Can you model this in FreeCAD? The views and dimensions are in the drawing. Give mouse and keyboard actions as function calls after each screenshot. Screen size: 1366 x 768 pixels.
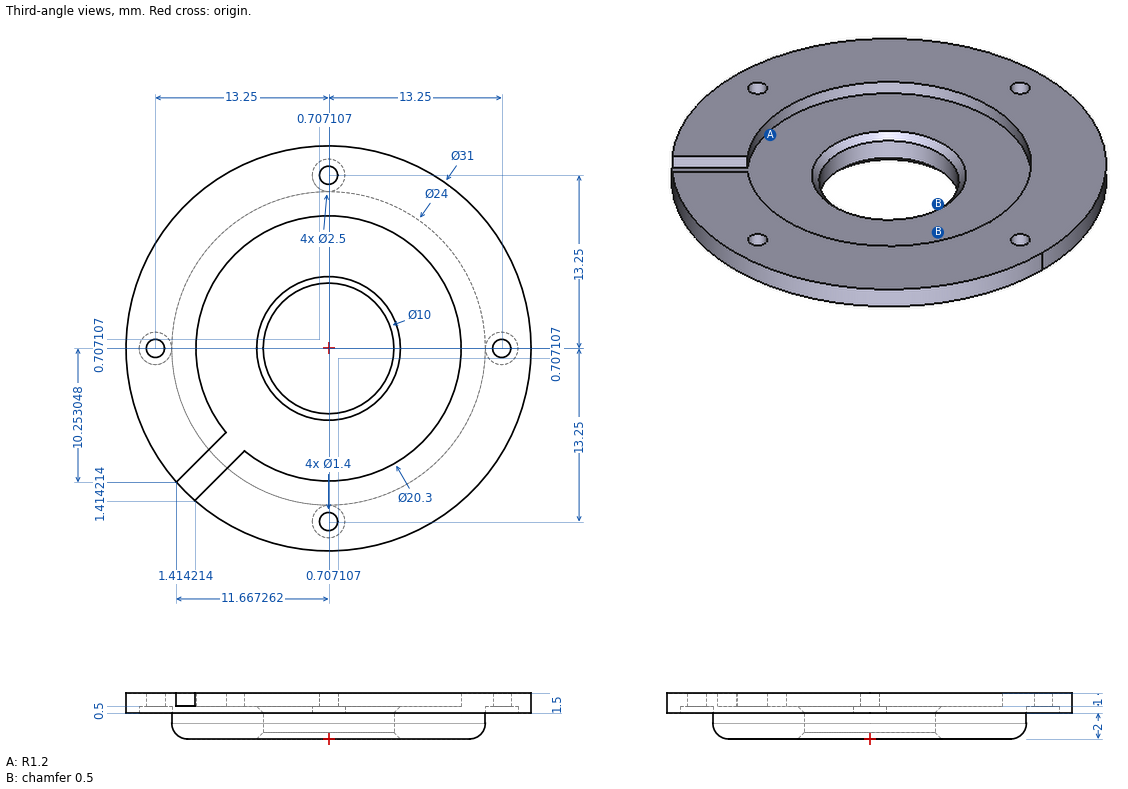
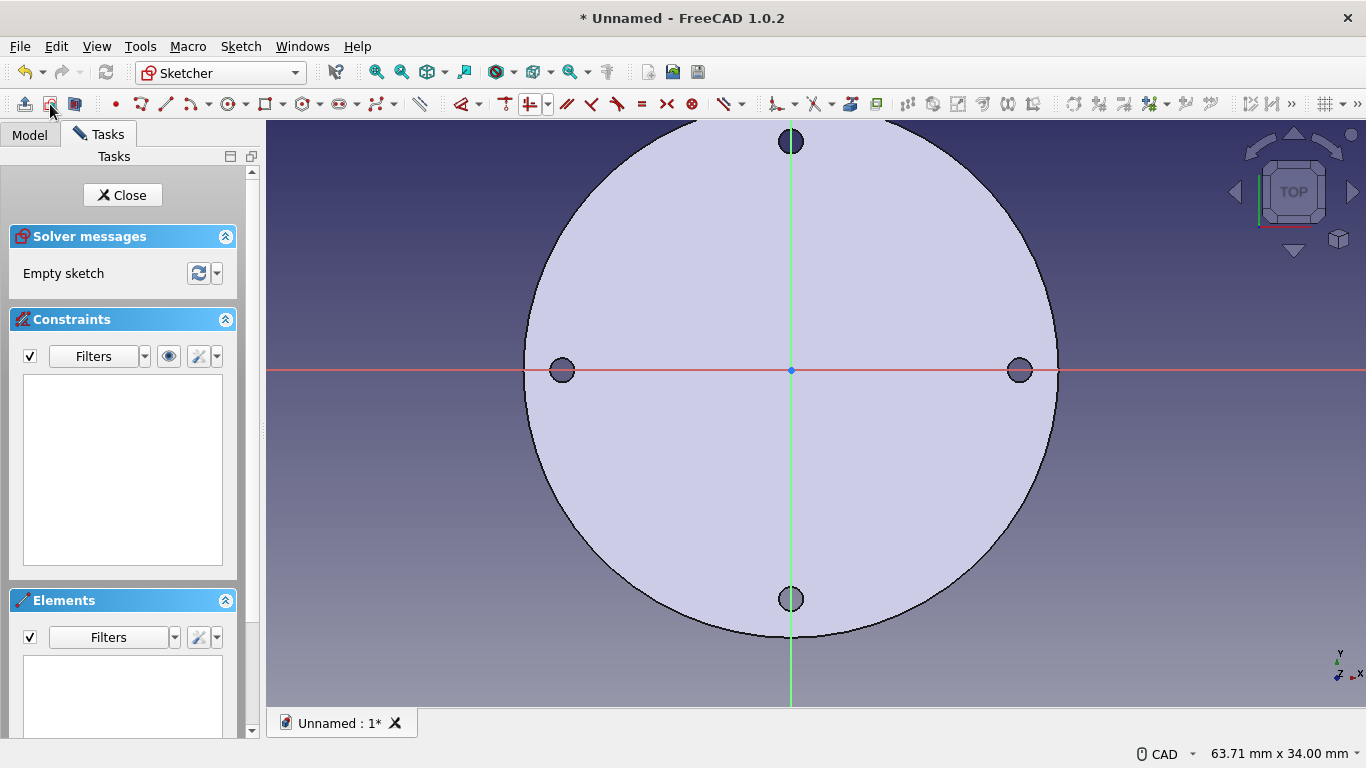
click(228, 104)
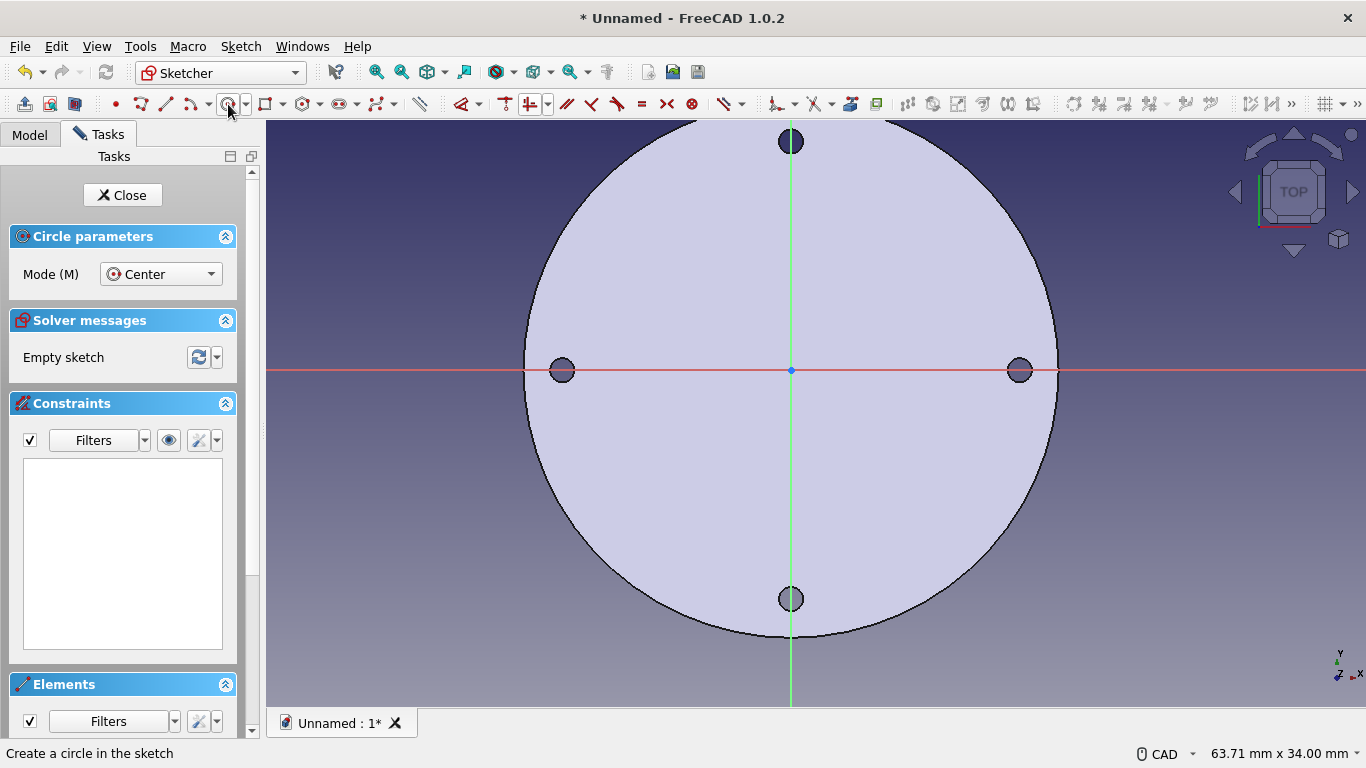
click(791, 370)
move(915, 246)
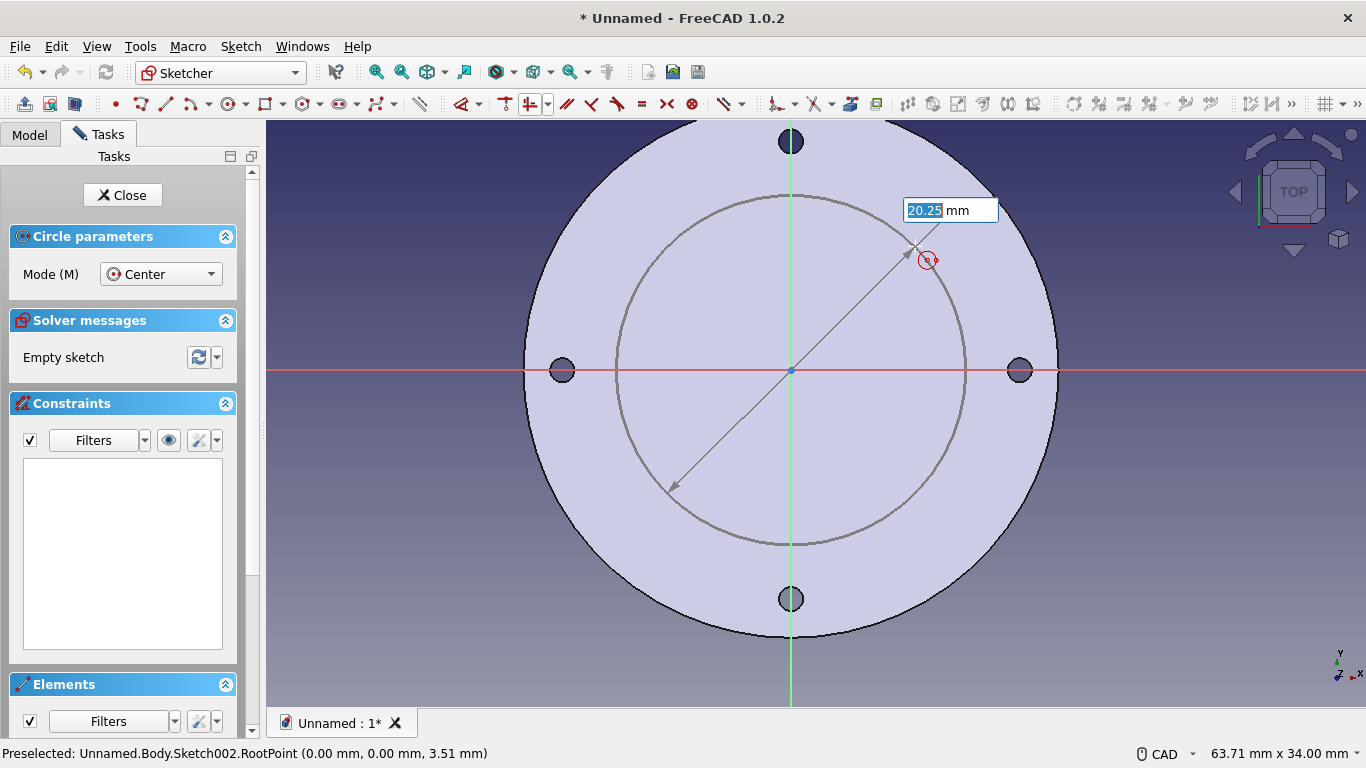
text(20.3)
key(Return)
key(Escape)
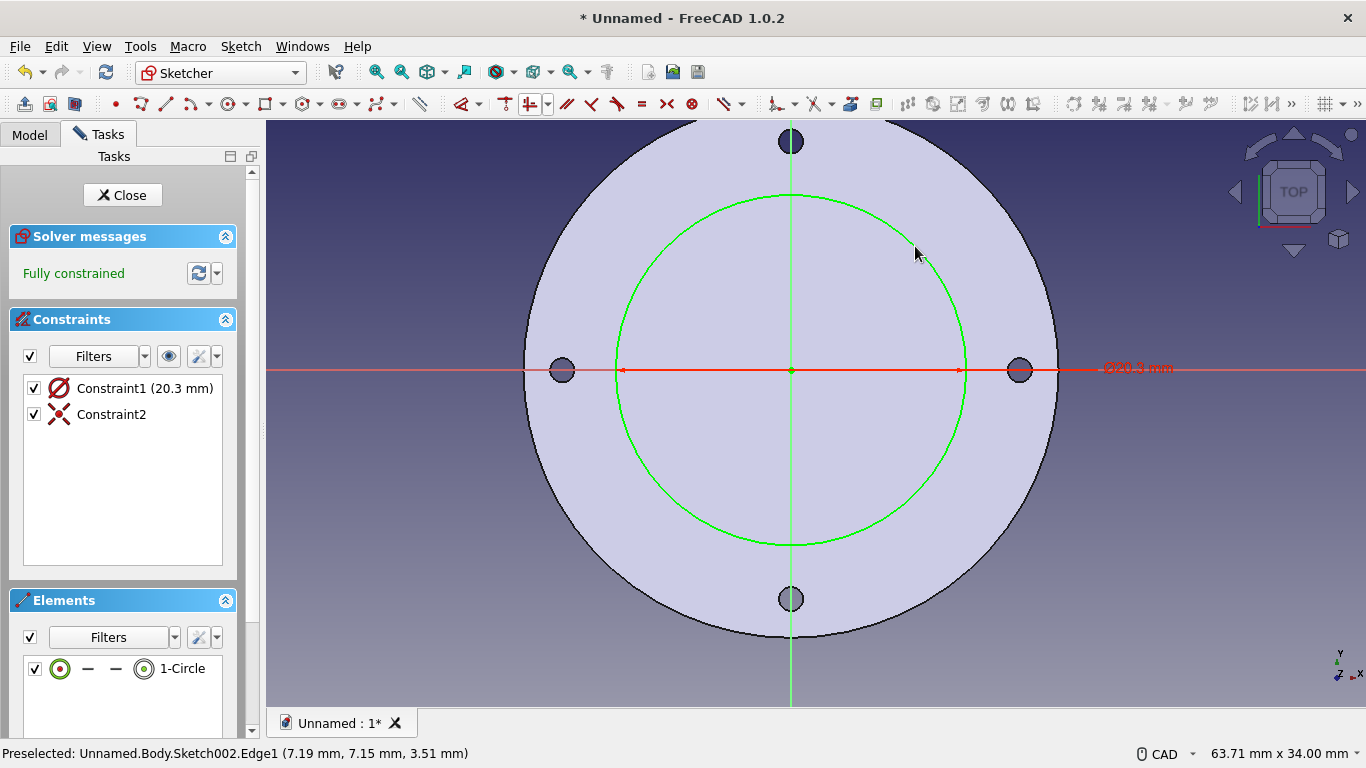
click(123, 195)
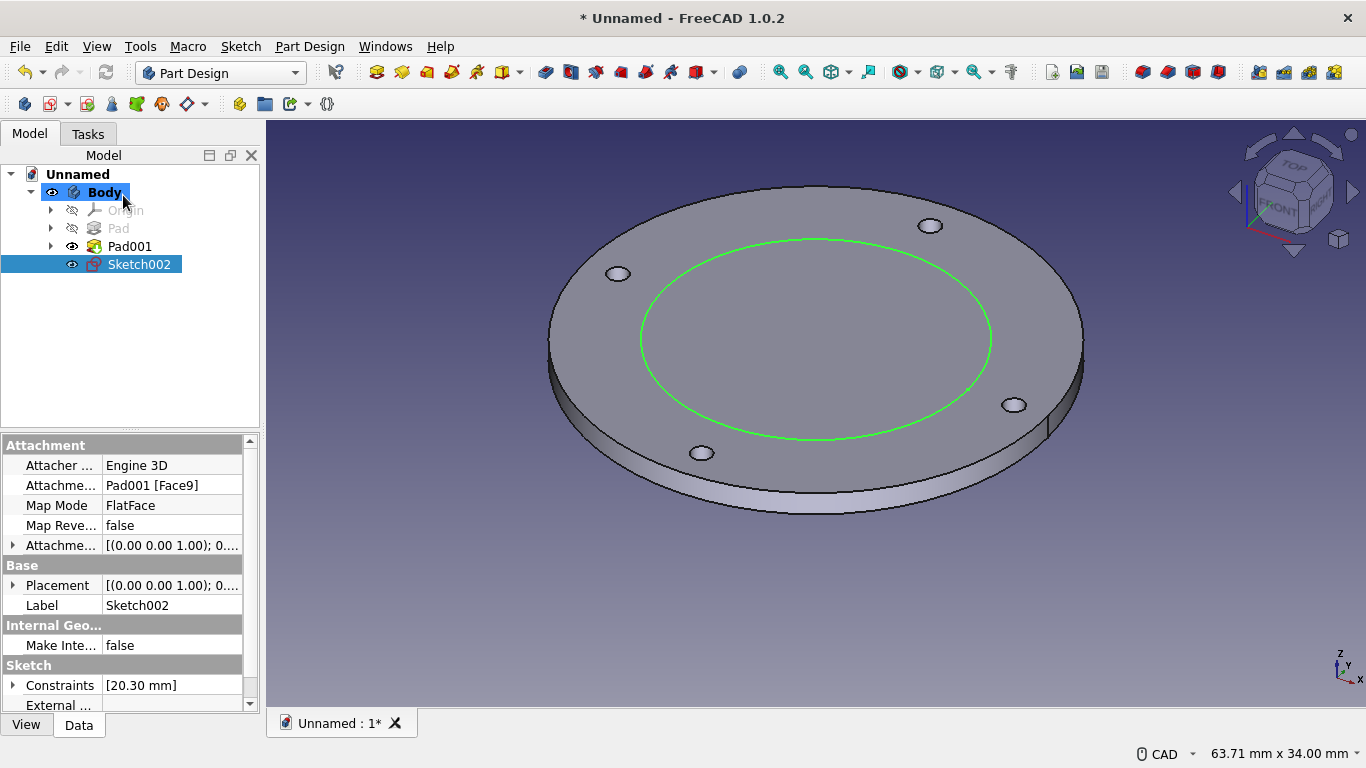
click(546, 72)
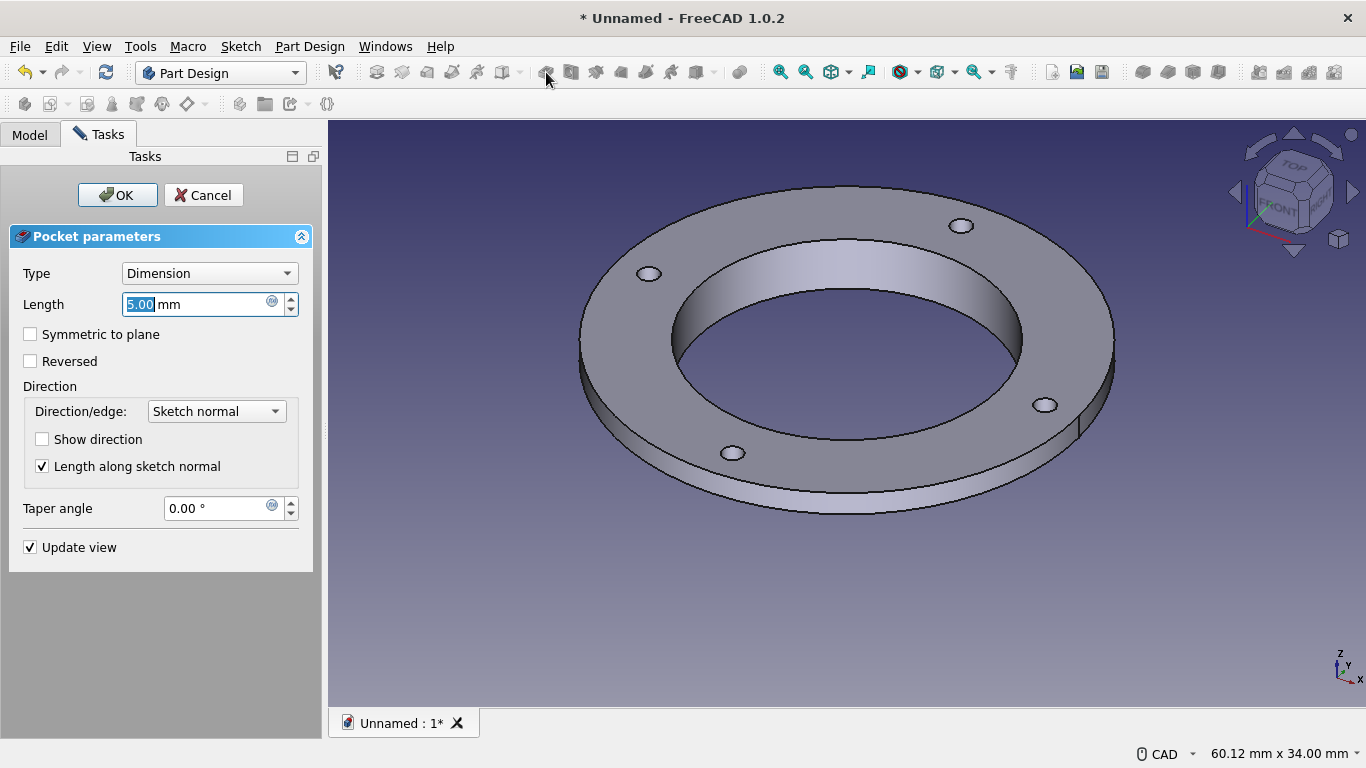
text(1)
key(Tab)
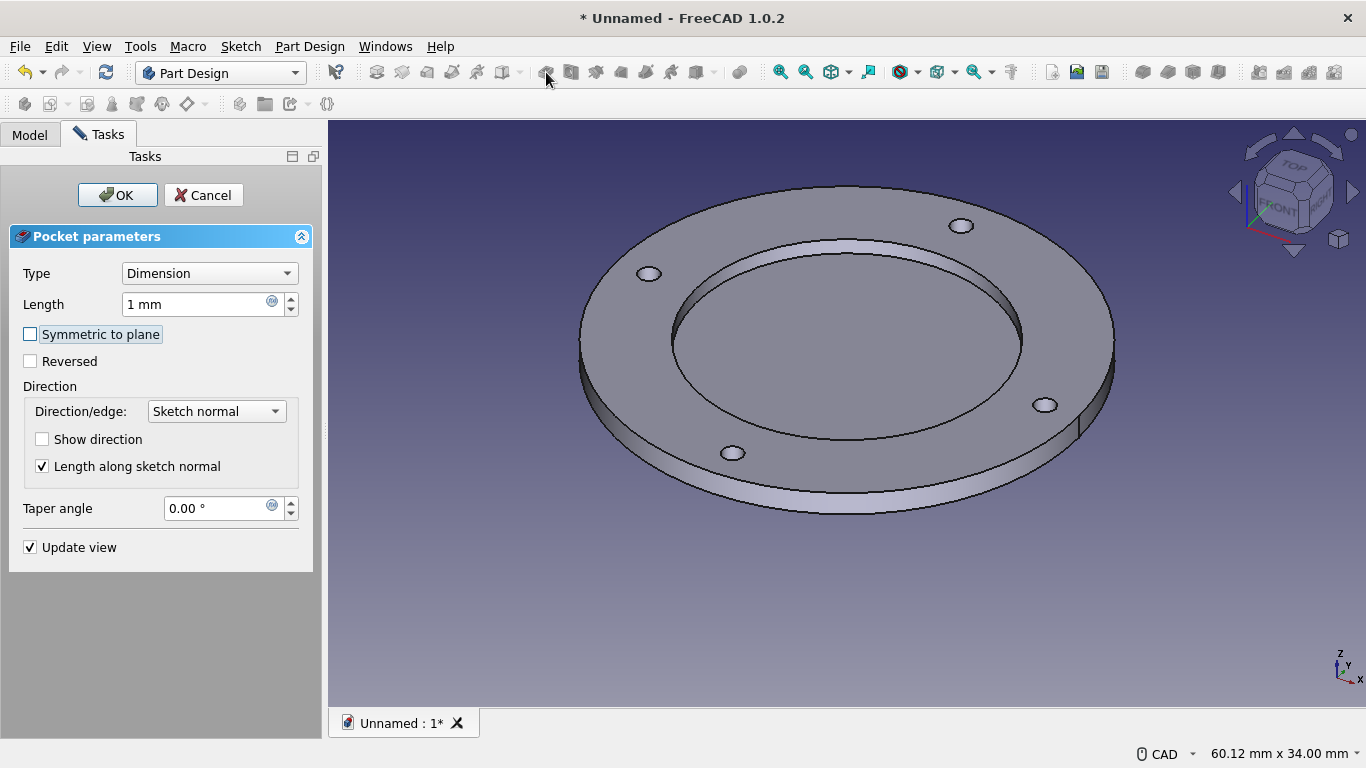
click(118, 195)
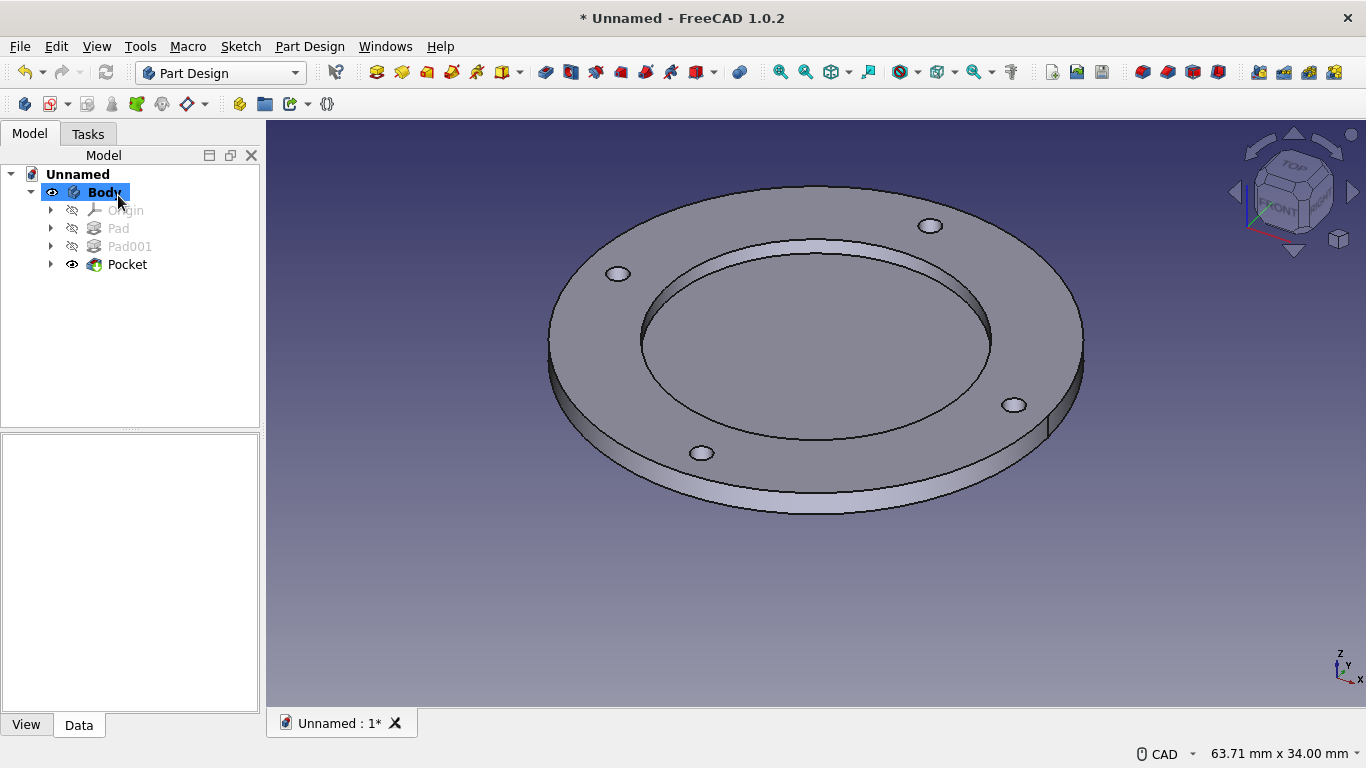
key(0)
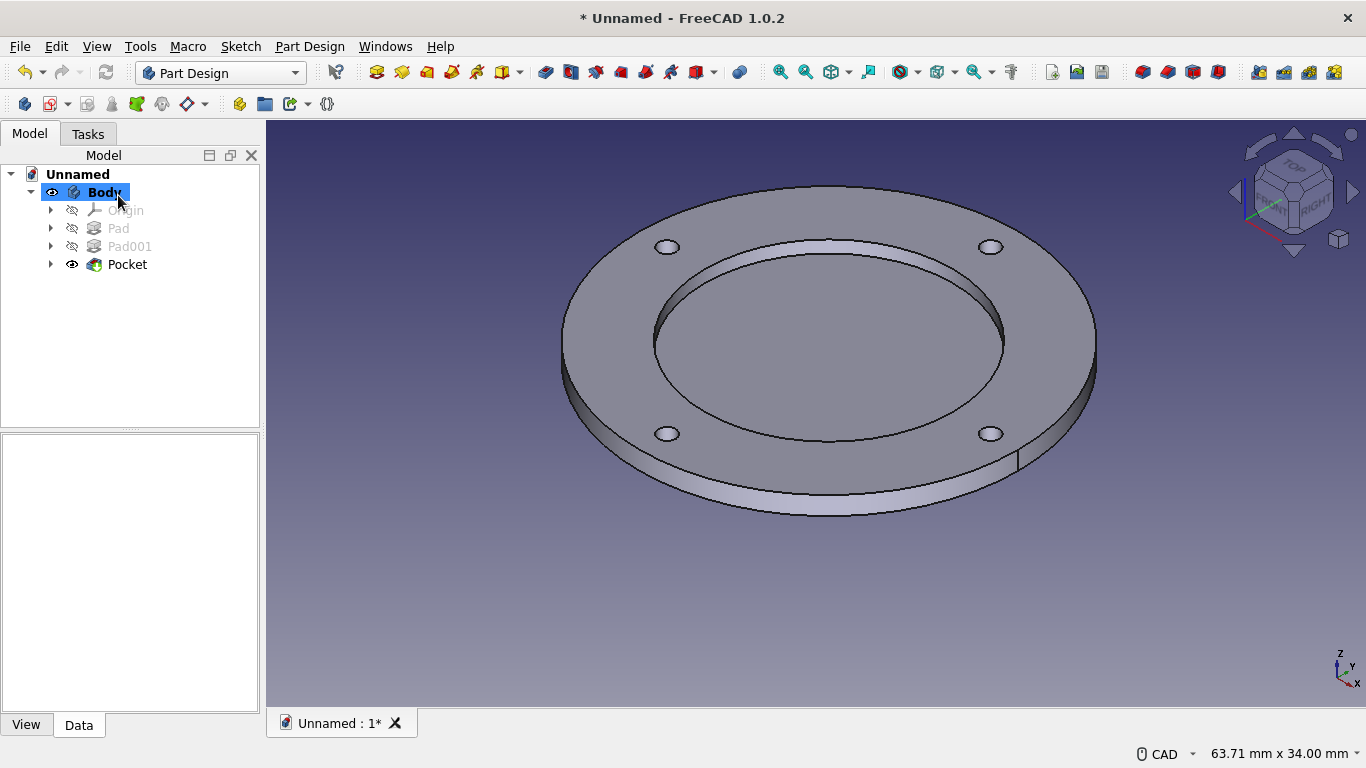
key(2)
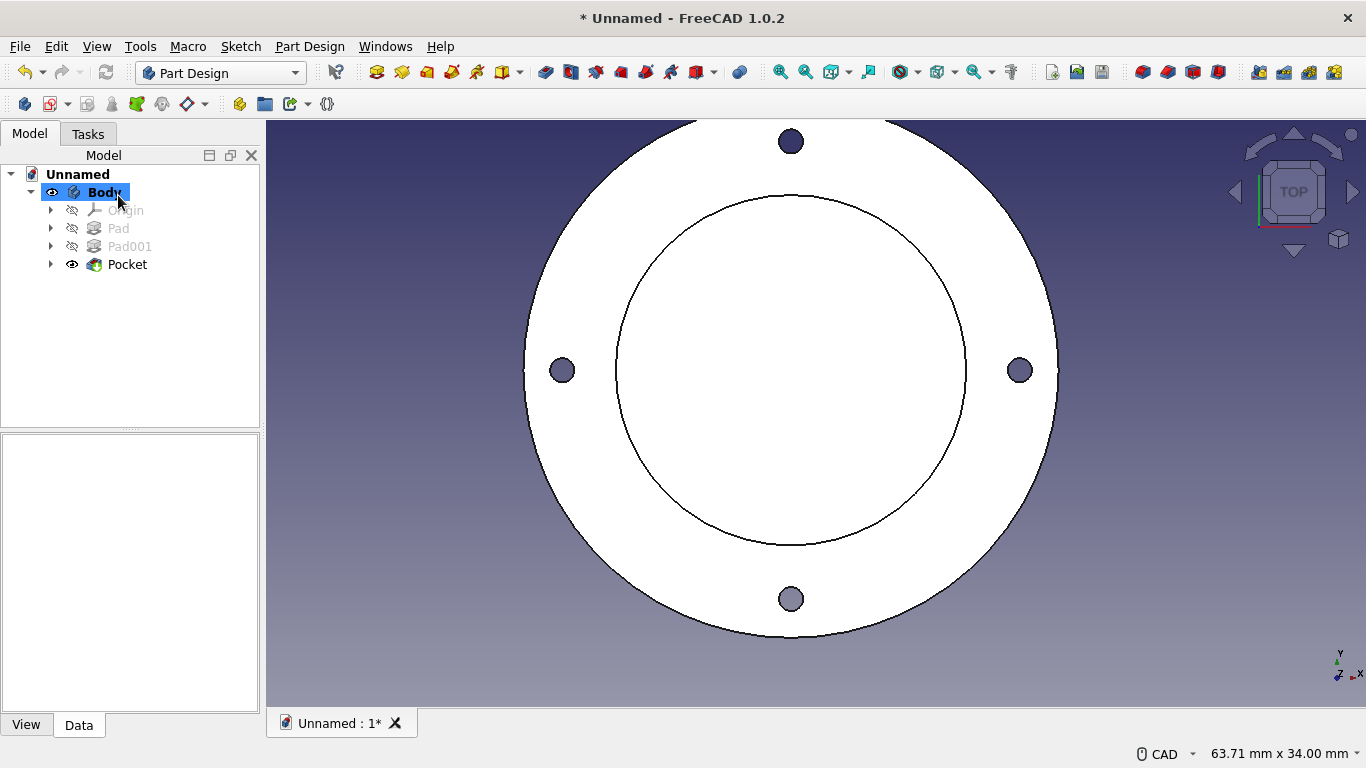
key(v)
key(f)